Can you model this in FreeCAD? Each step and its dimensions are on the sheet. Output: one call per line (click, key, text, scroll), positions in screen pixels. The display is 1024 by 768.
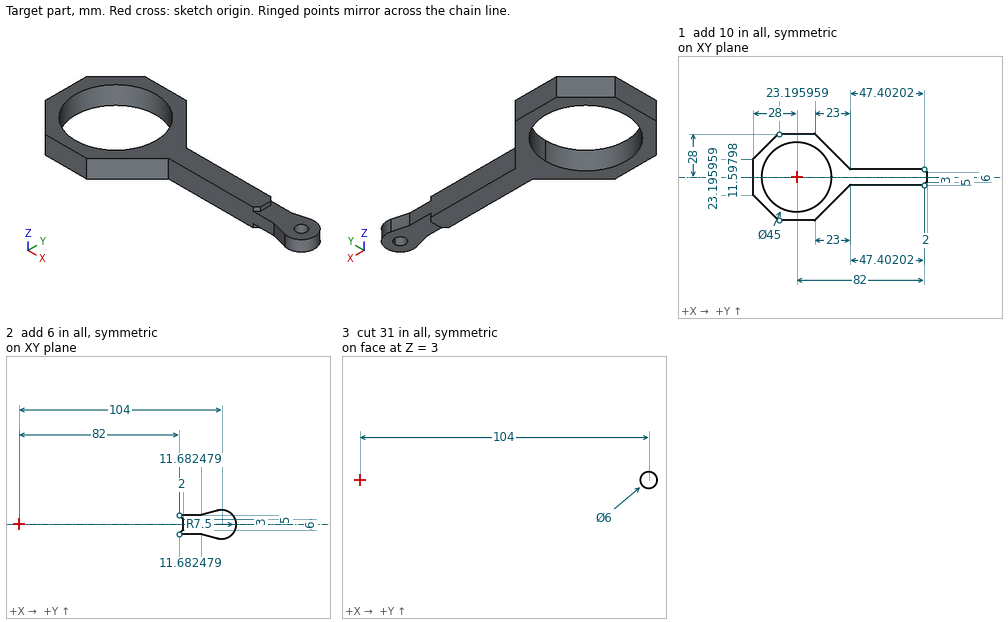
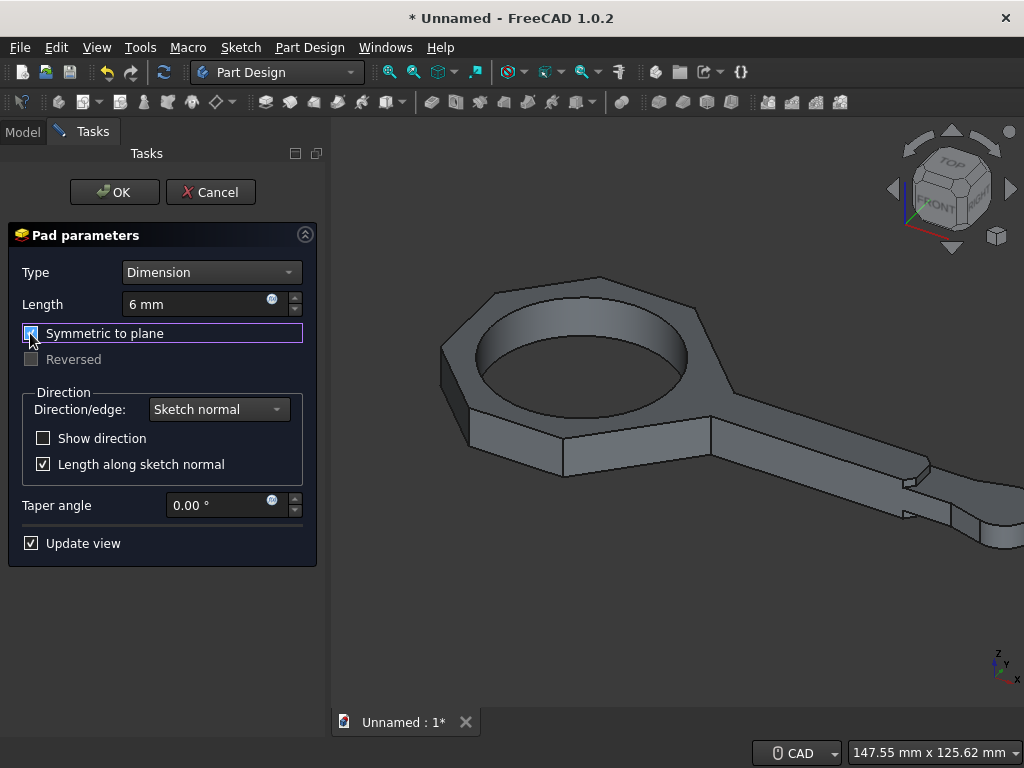
click(115, 192)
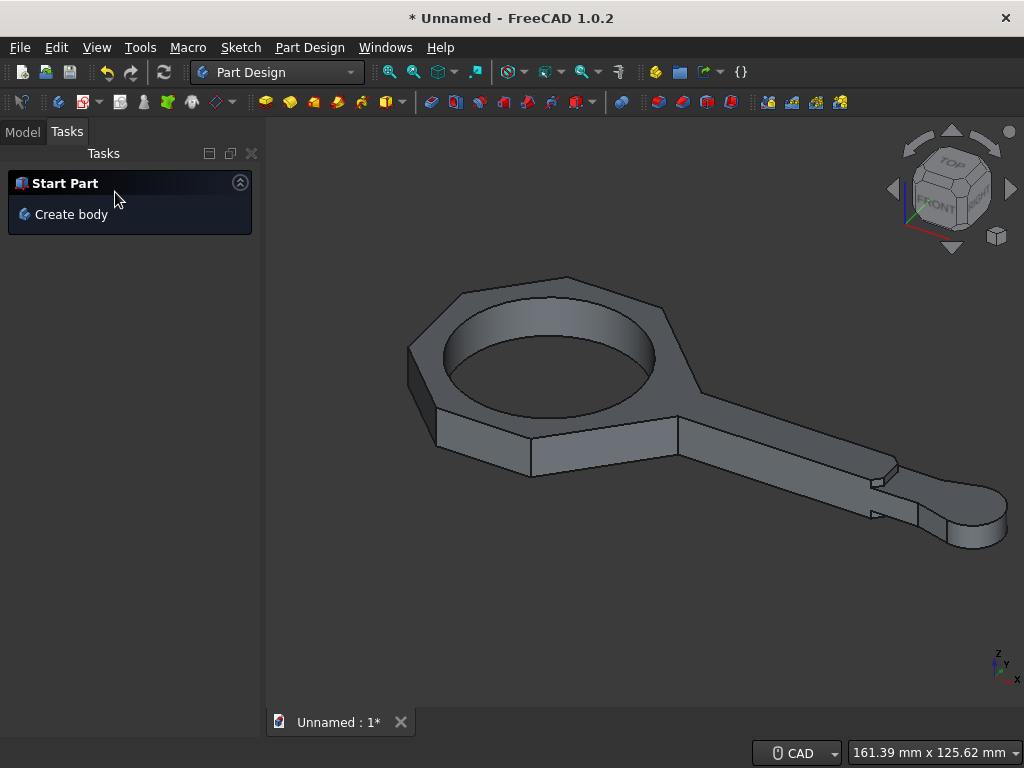
click(390, 72)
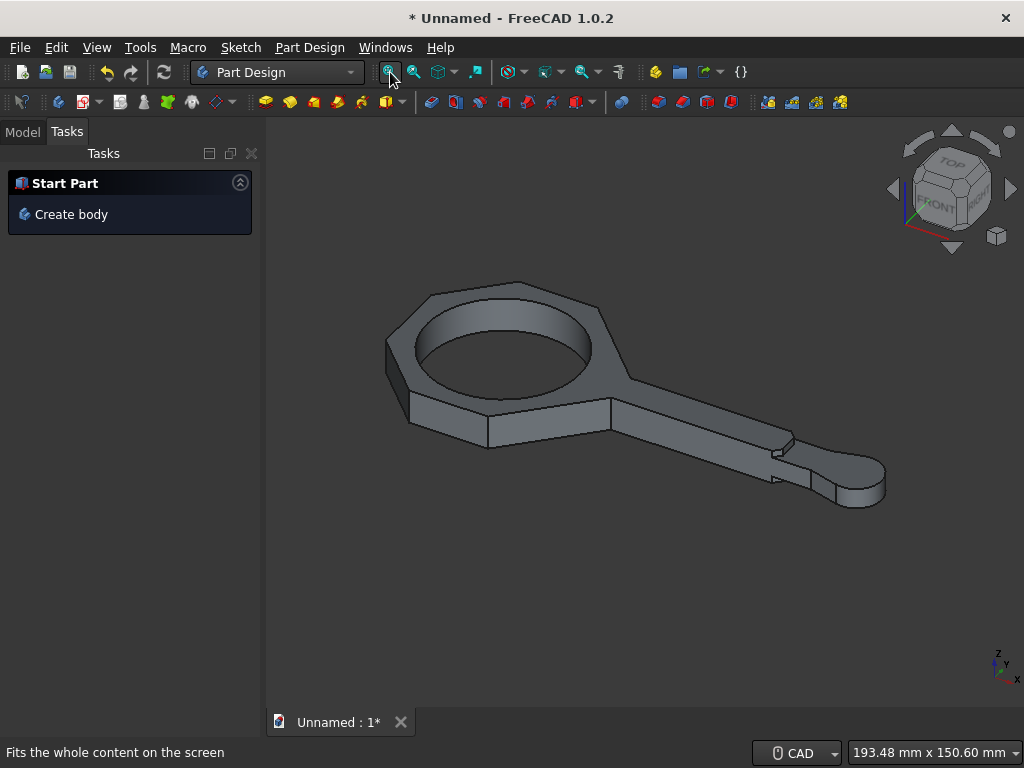
click(846, 468)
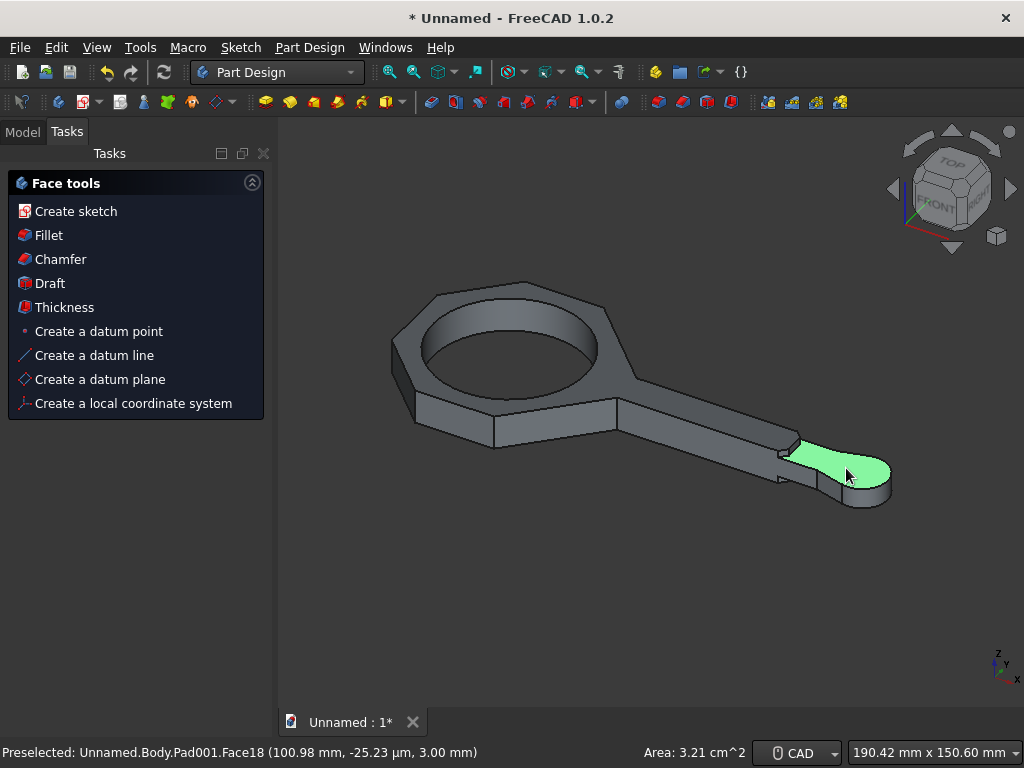
click(84, 102)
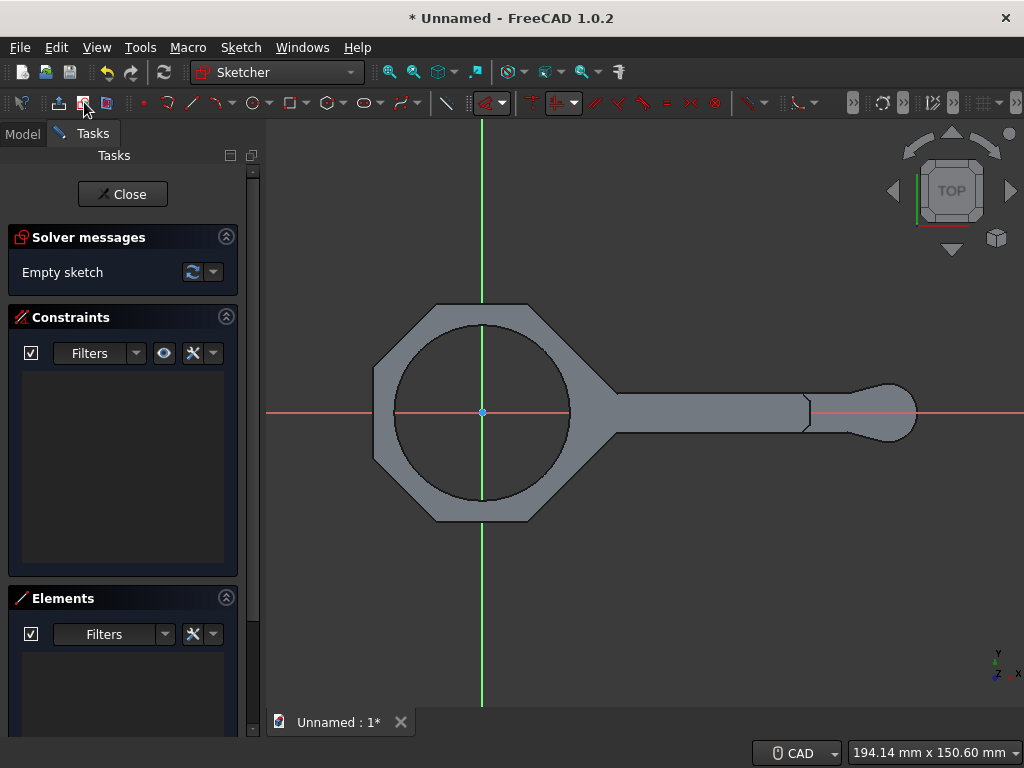
scroll(576, 413, down, 5)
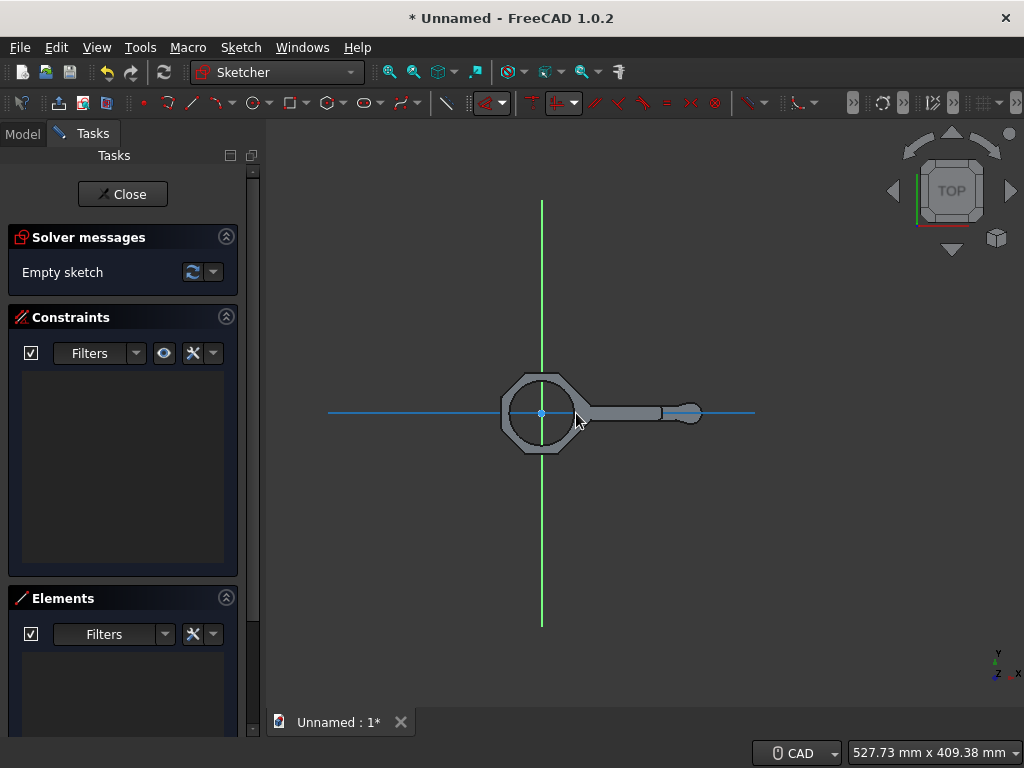
scroll(697, 413, up, 15)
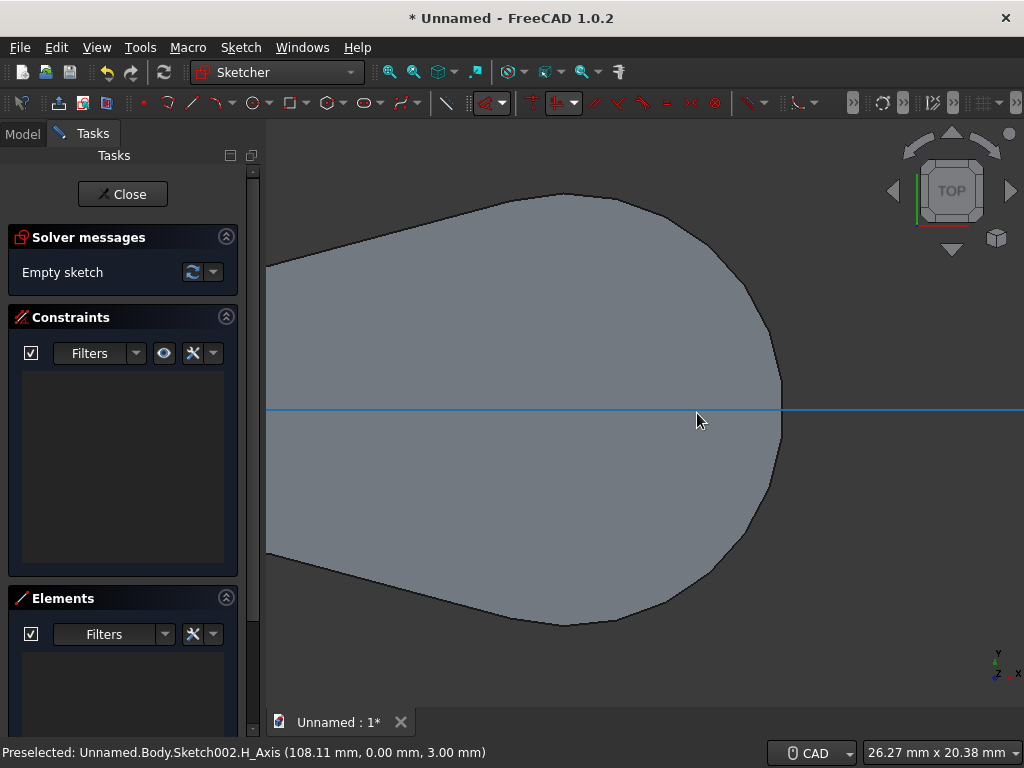
scroll(560, 407, up, 4)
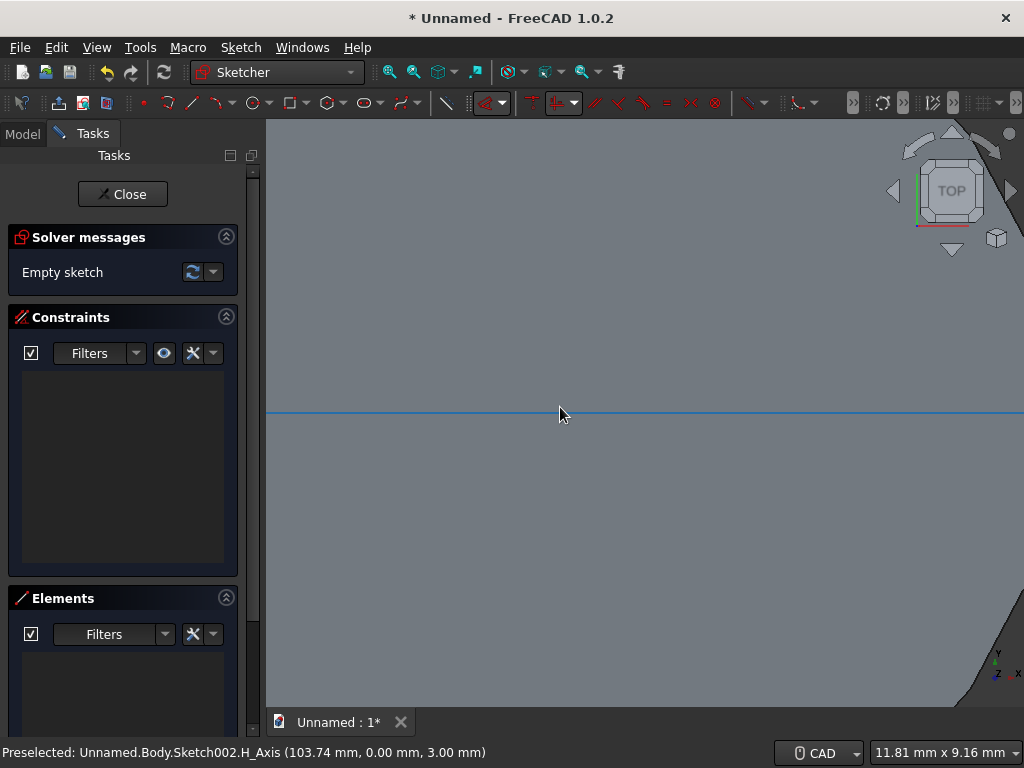
click(254, 104)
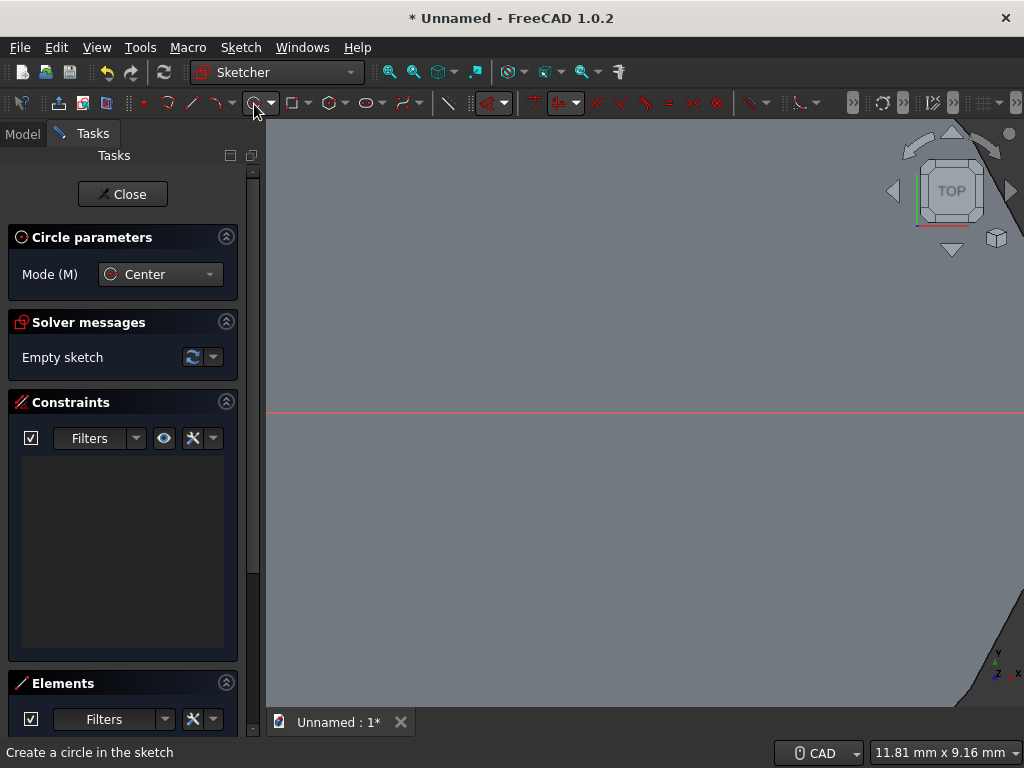
click(576, 413)
move(712, 276)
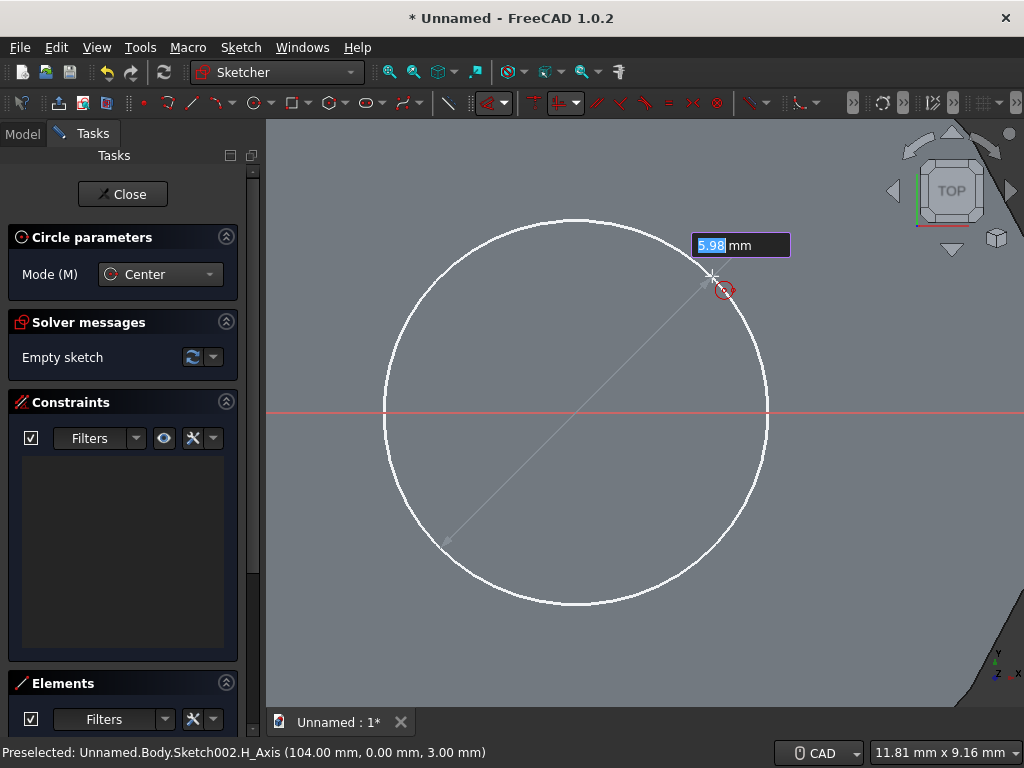
text(6)
key(Return)
key(Escape)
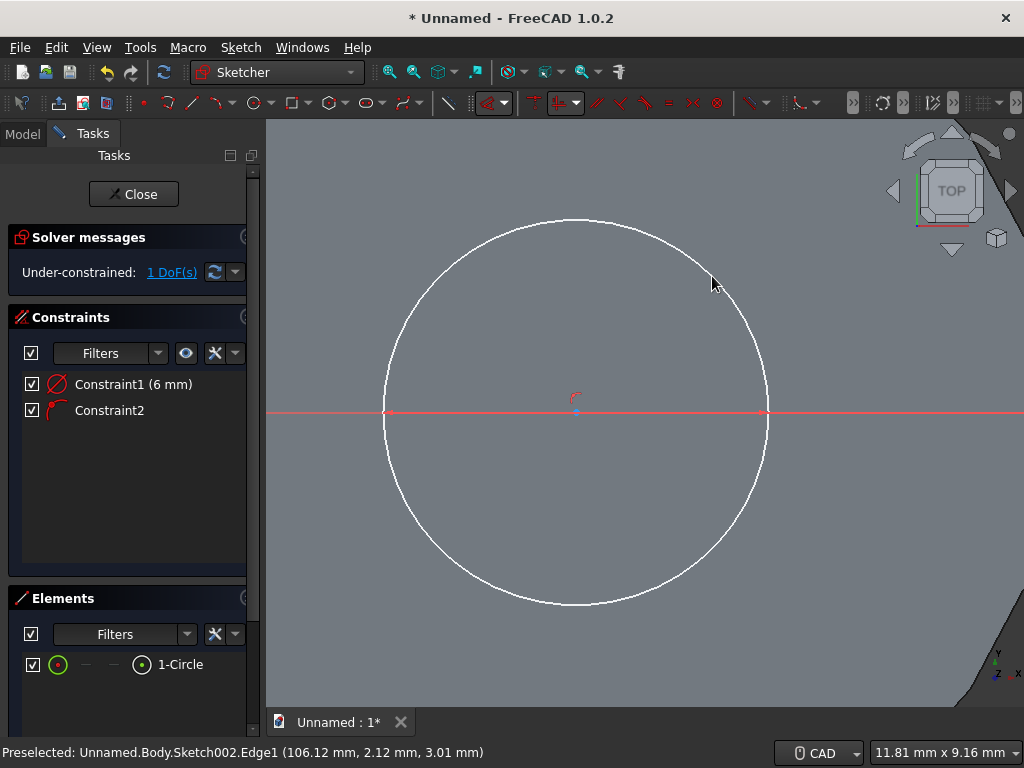
click(576, 413)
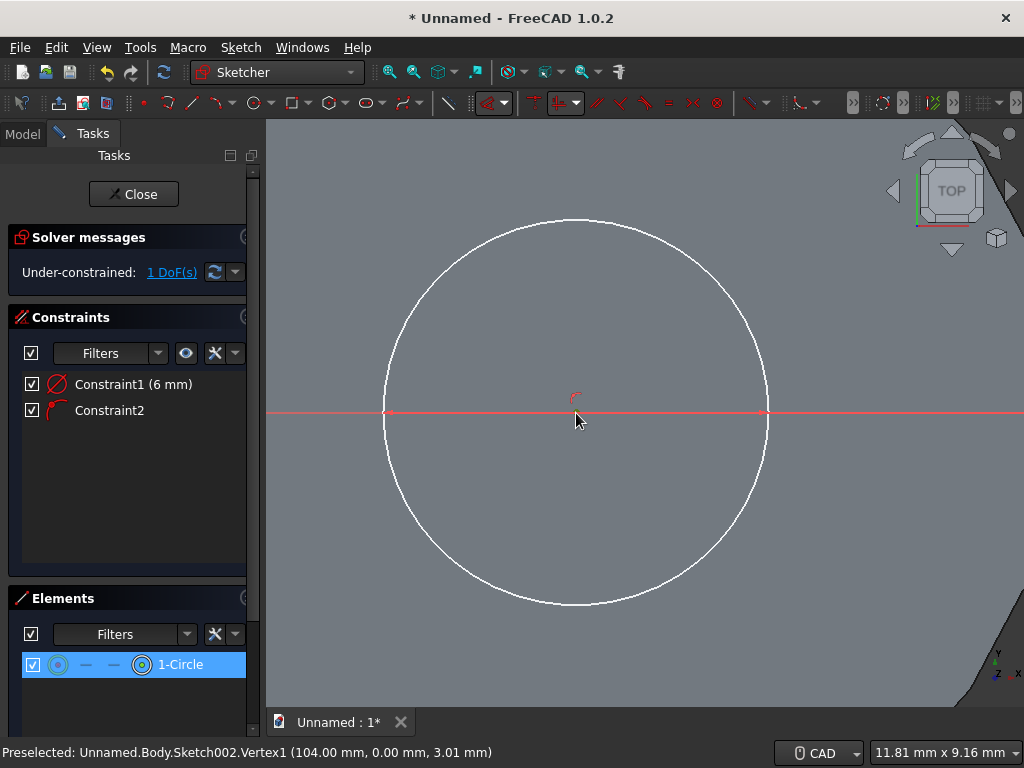
key(l)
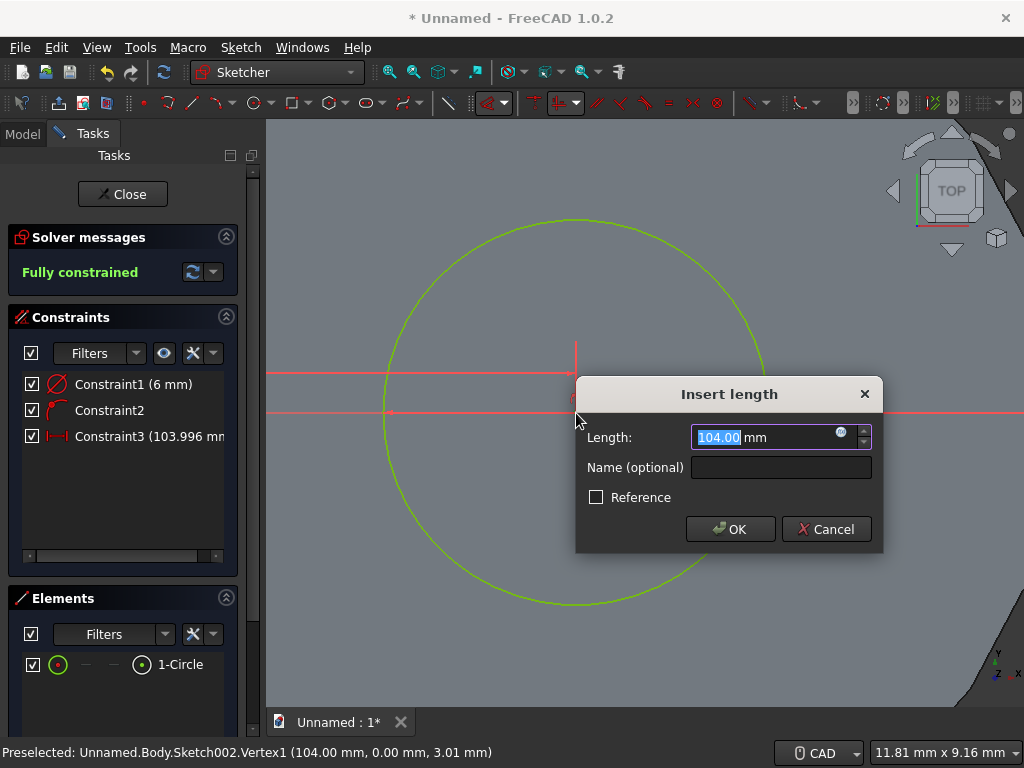
text(104)
key(Return)